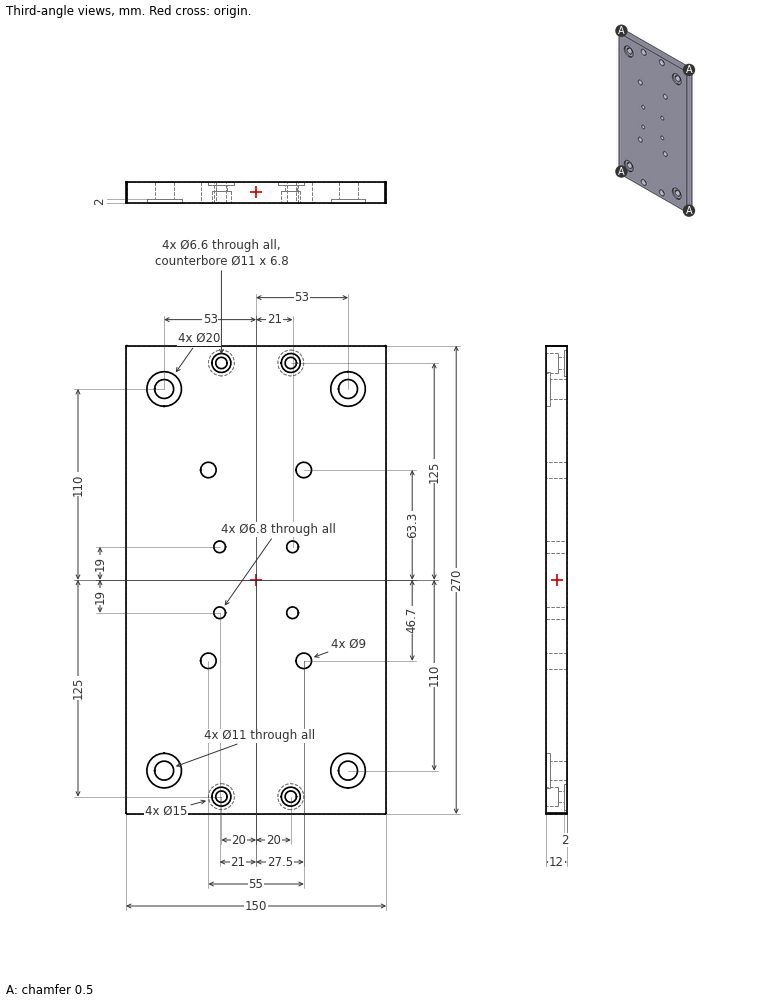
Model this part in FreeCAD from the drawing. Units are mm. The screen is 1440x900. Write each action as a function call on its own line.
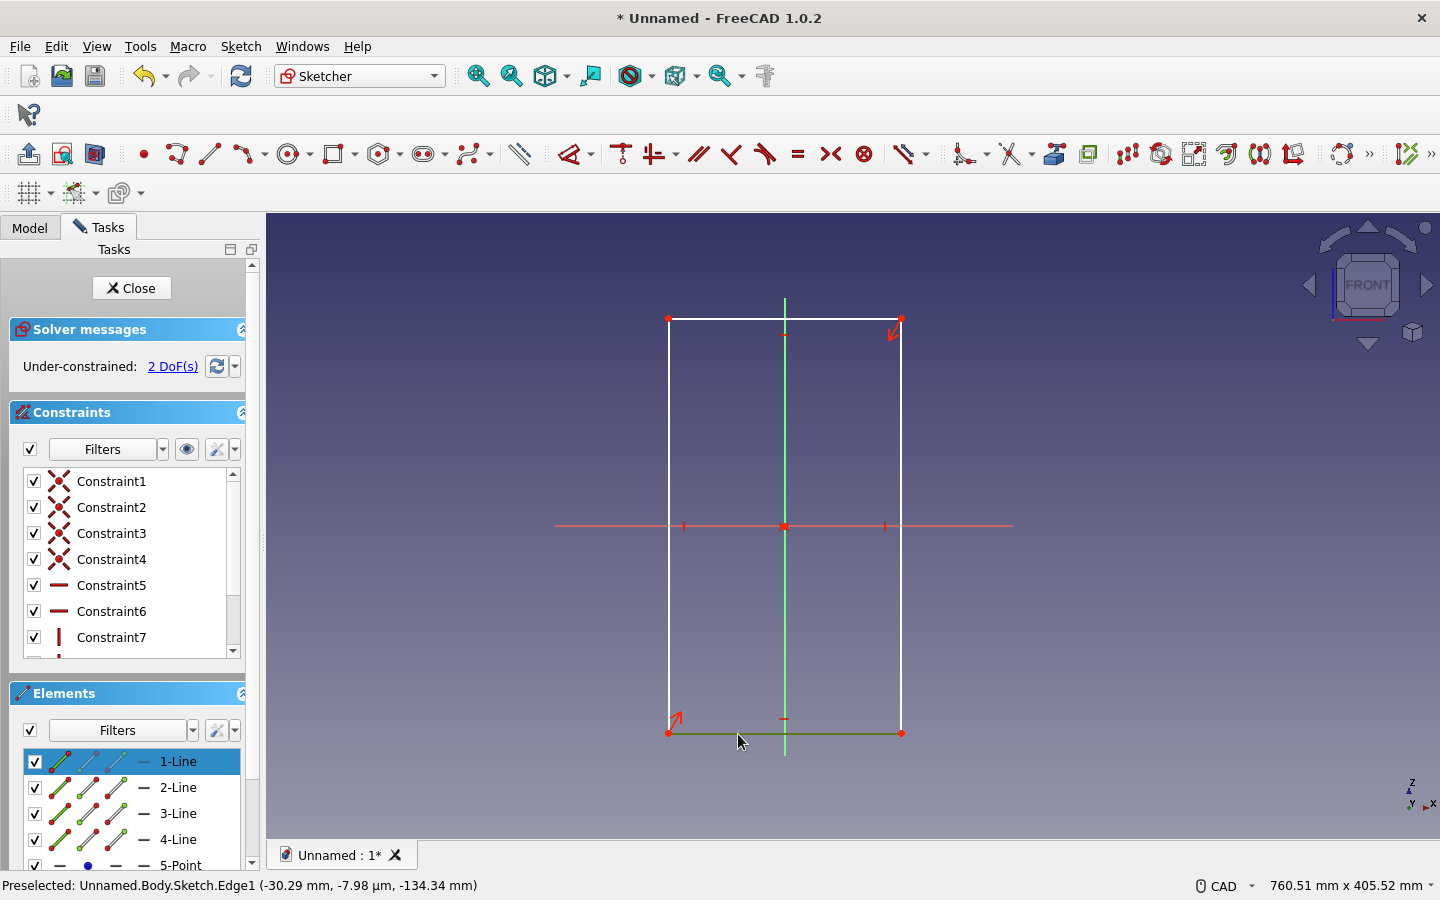
key(l)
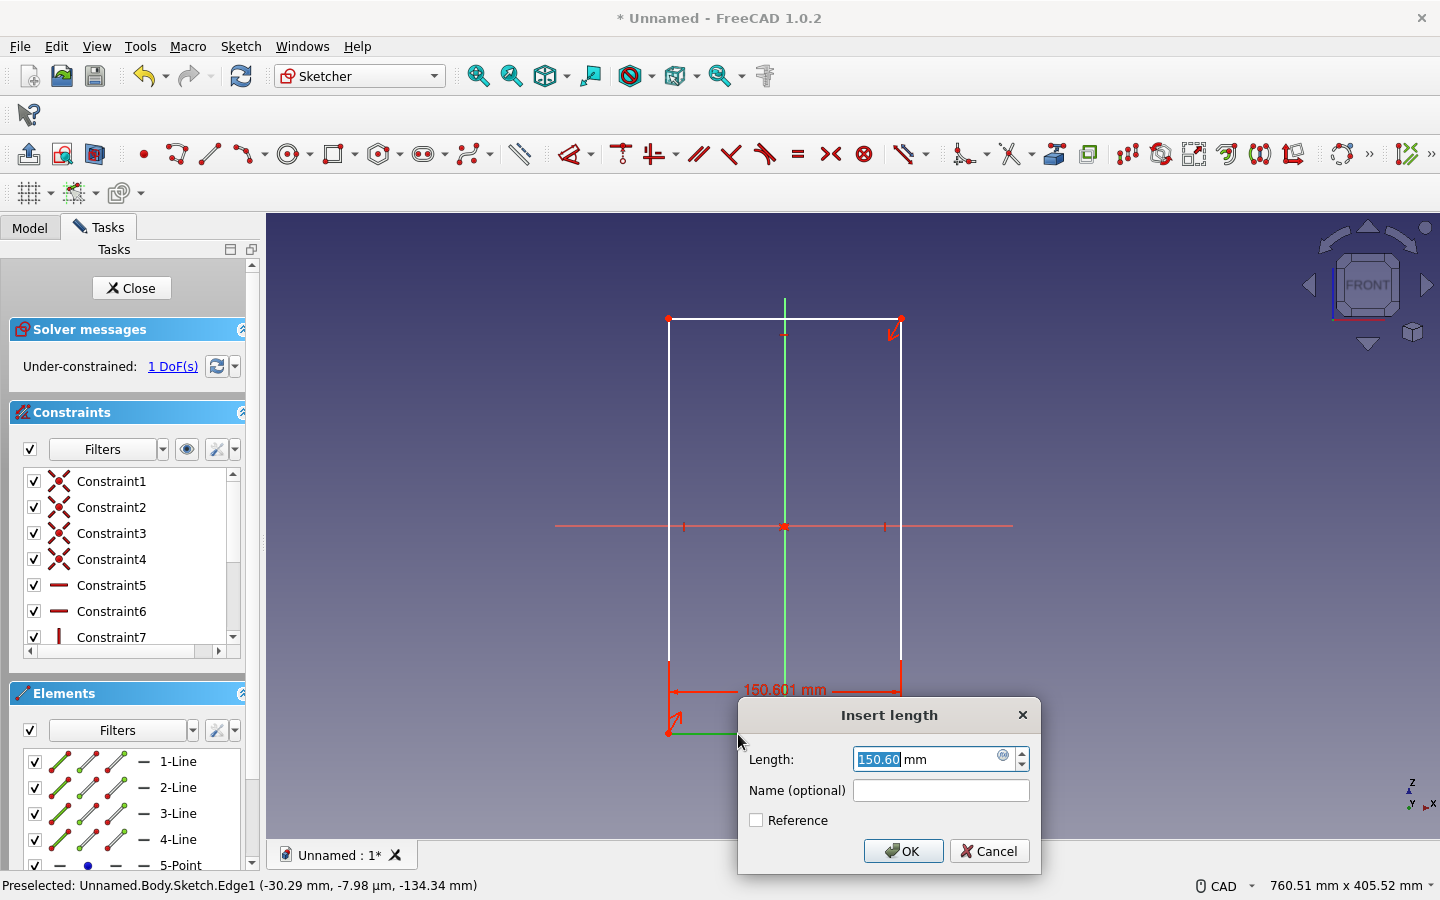
text(150)
key(Return)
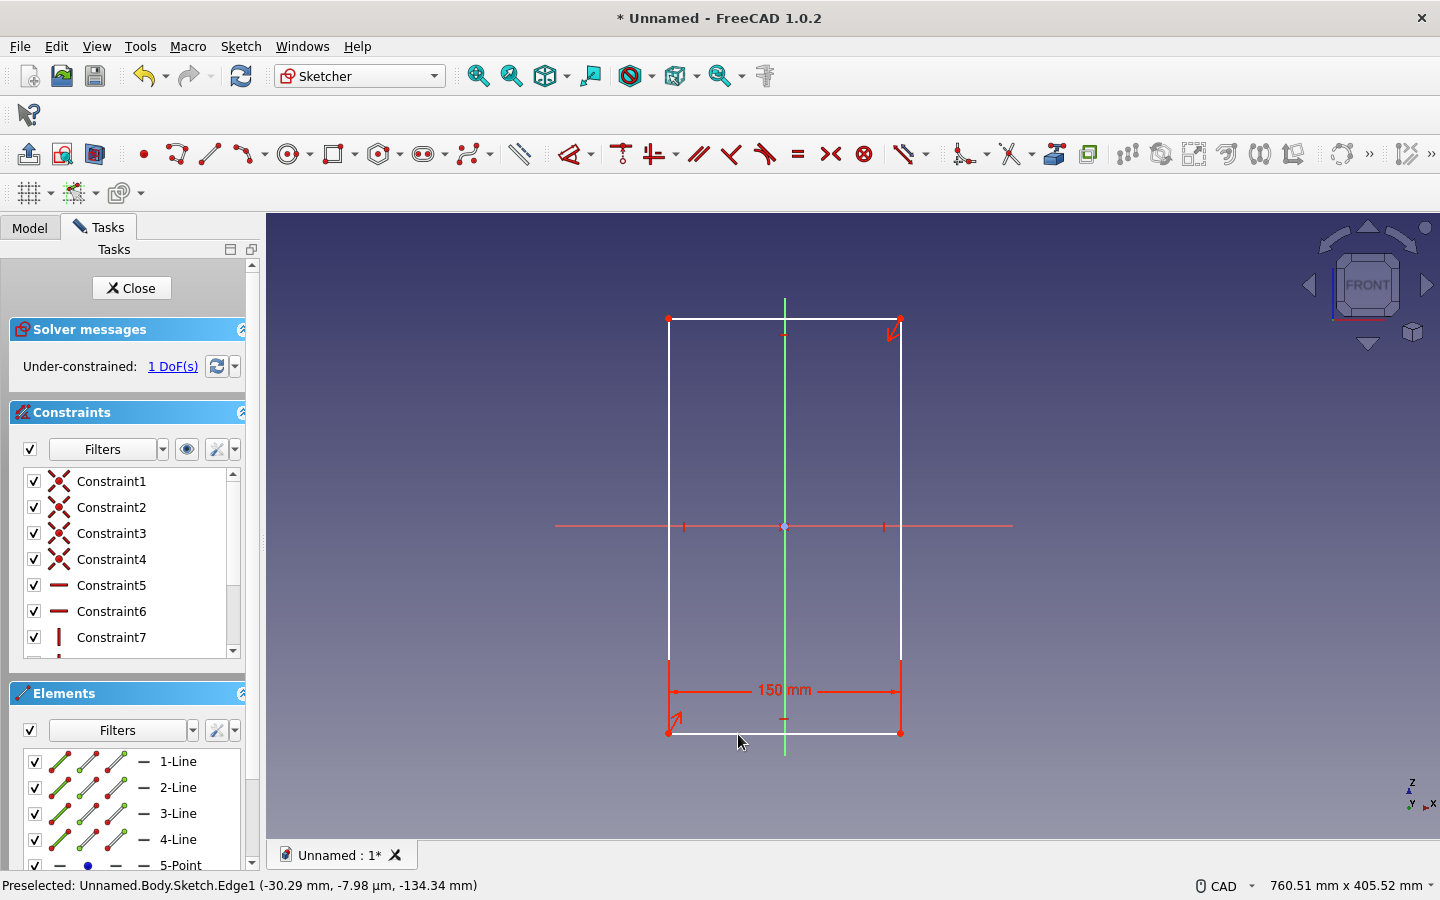
click(901, 609)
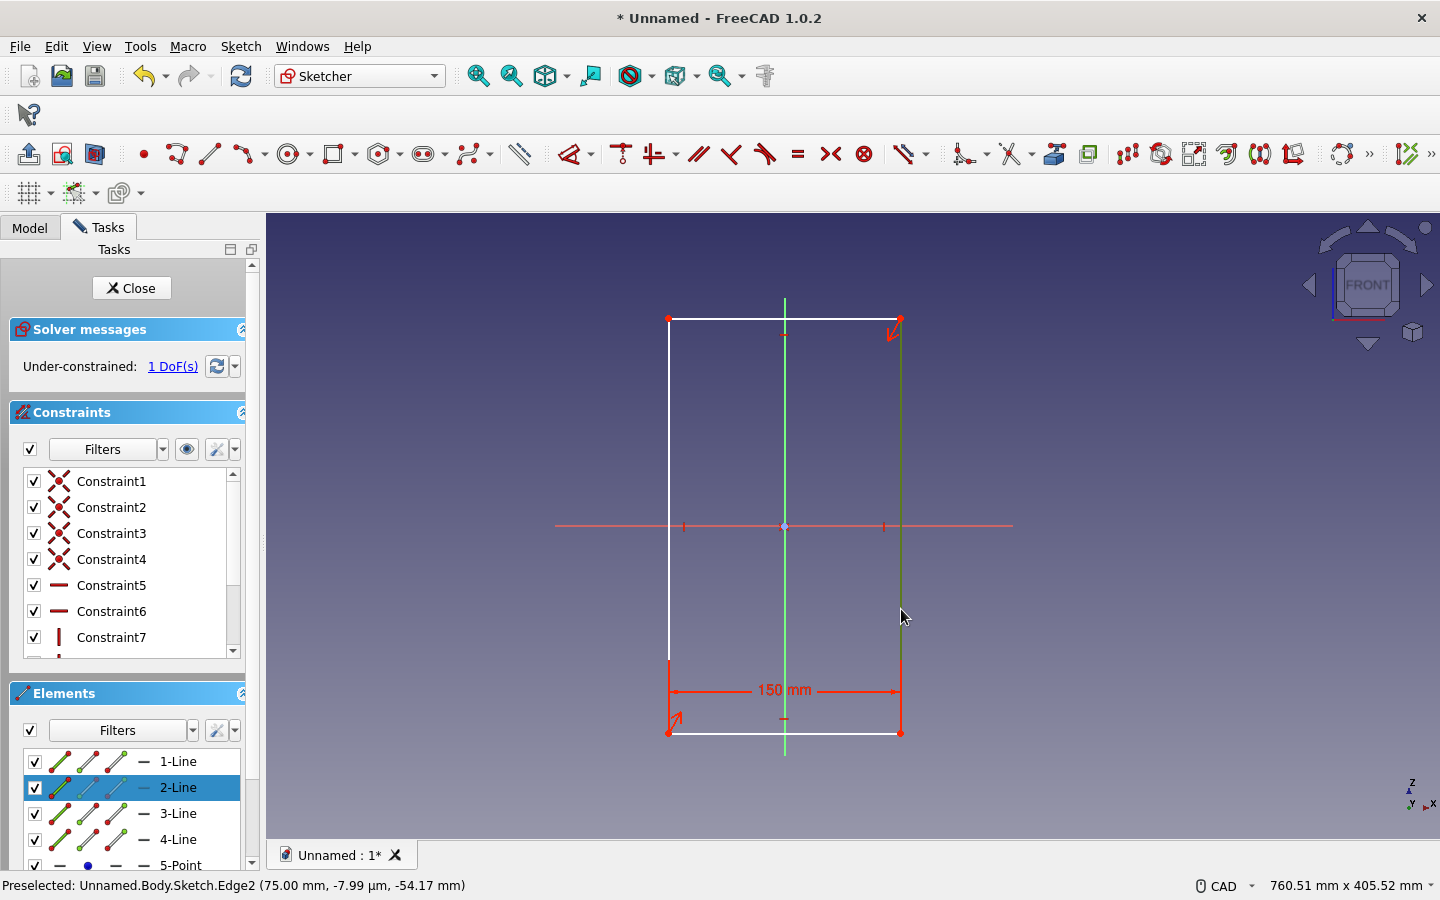
click(590, 154)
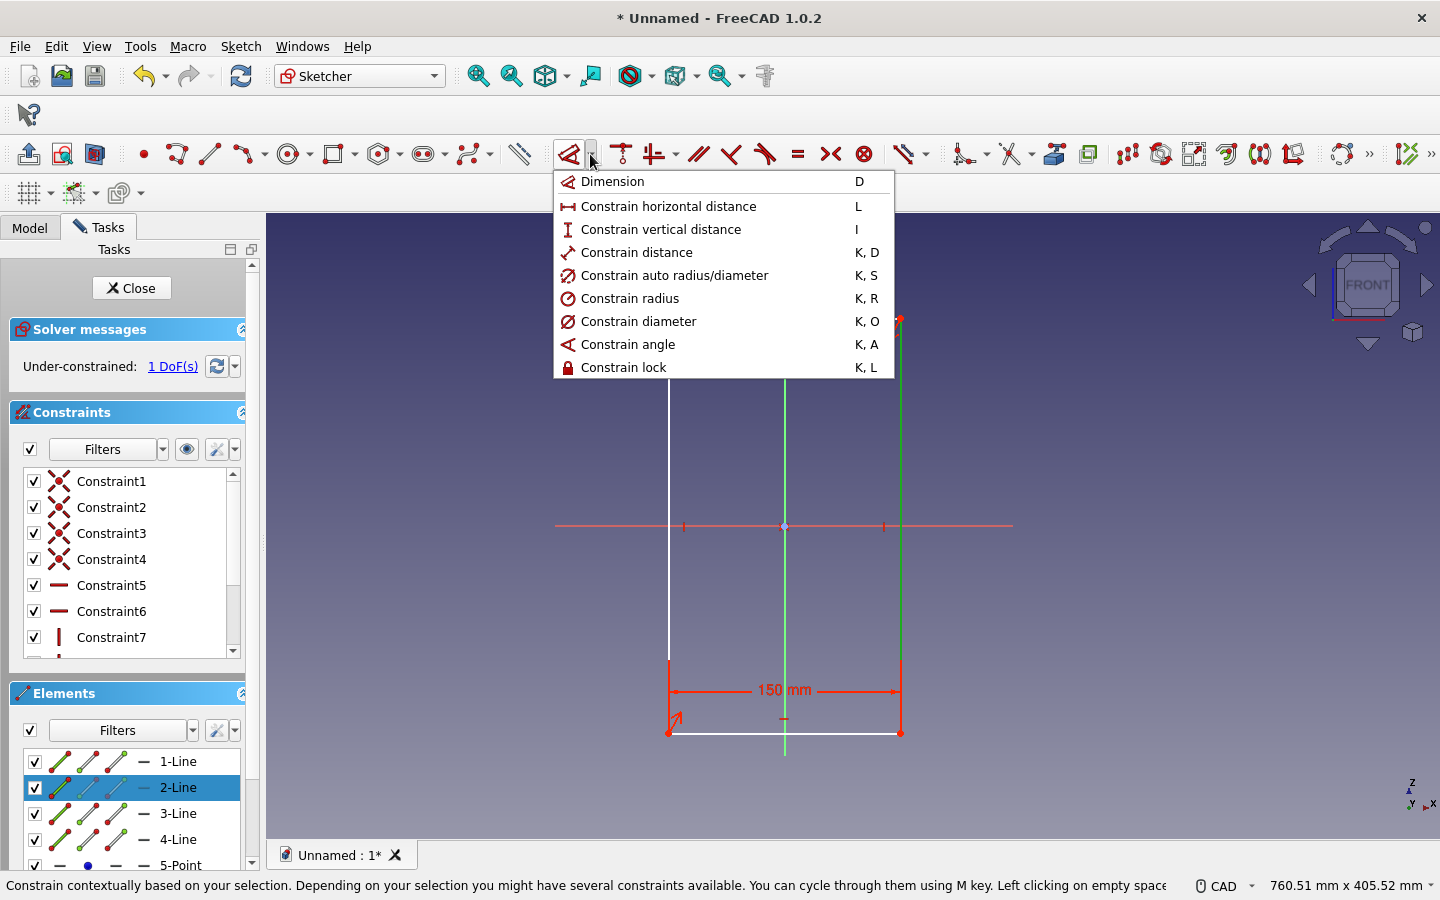
click(724, 230)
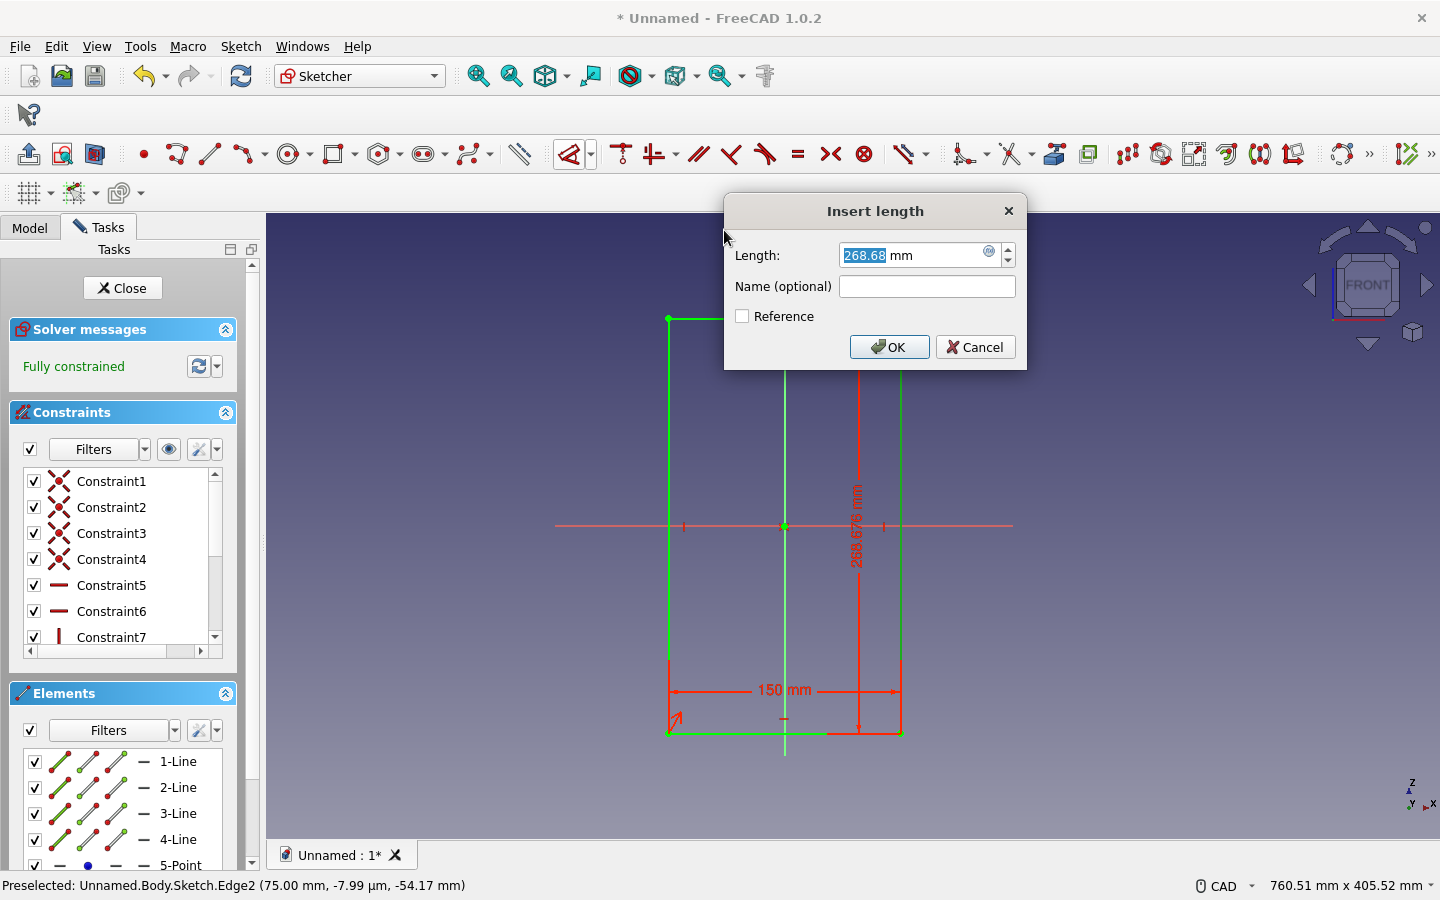
text(270)
key(Return)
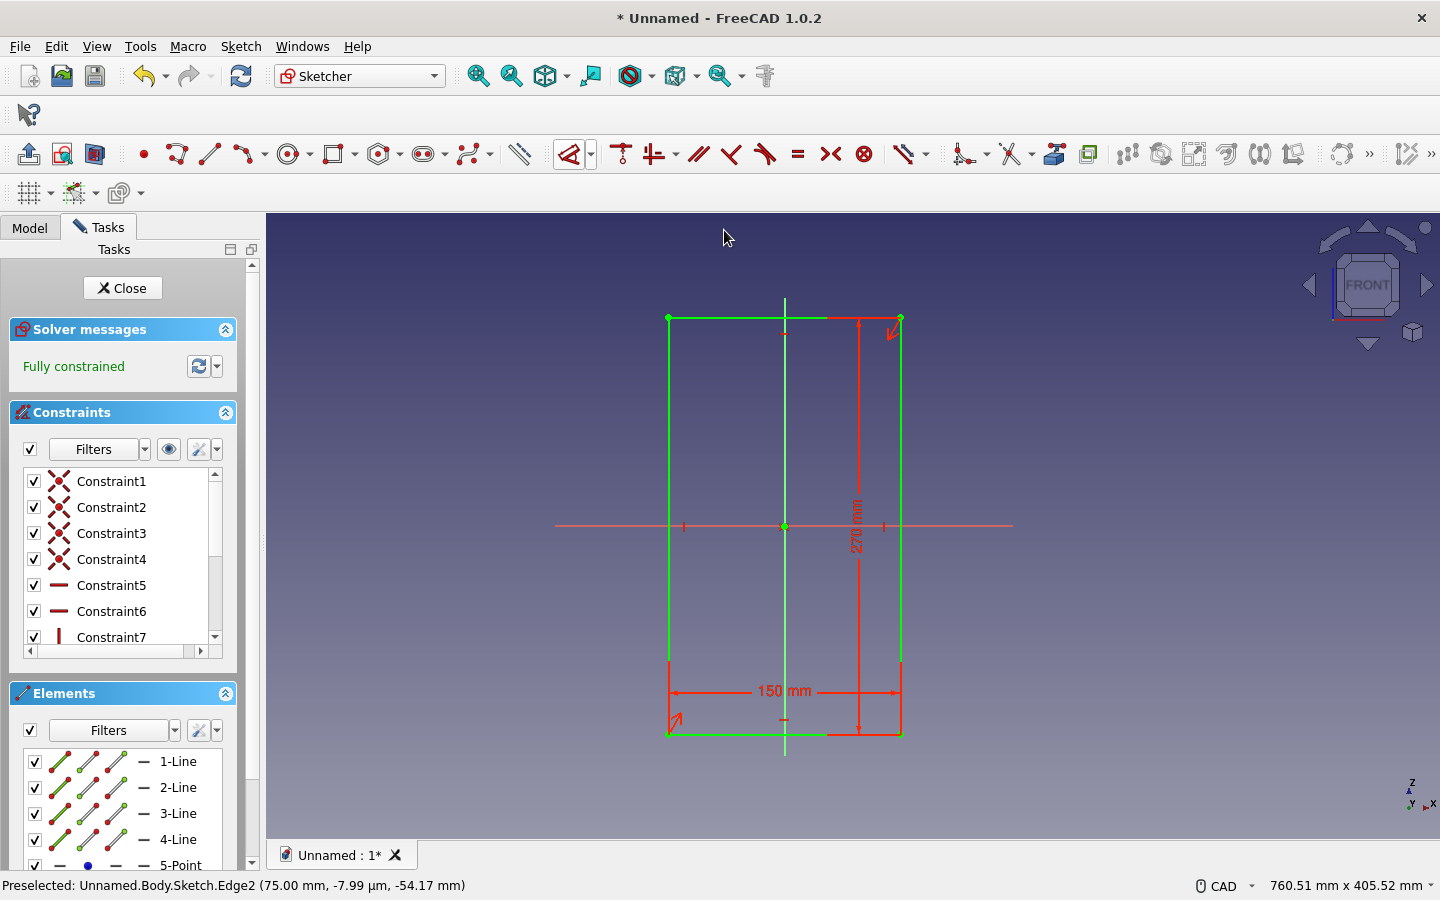
click(123, 288)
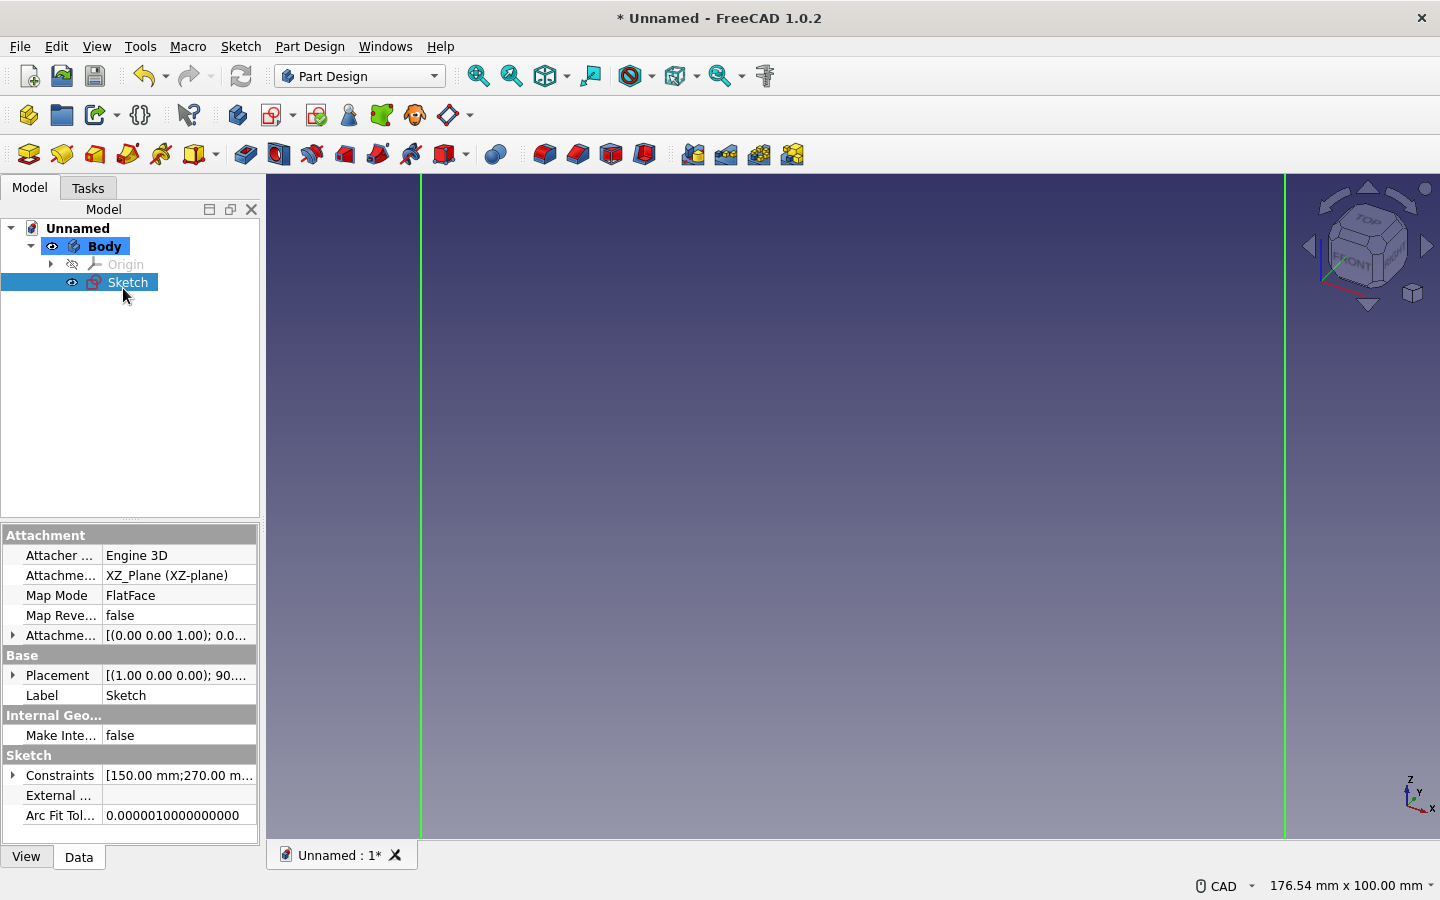
click(29, 154)